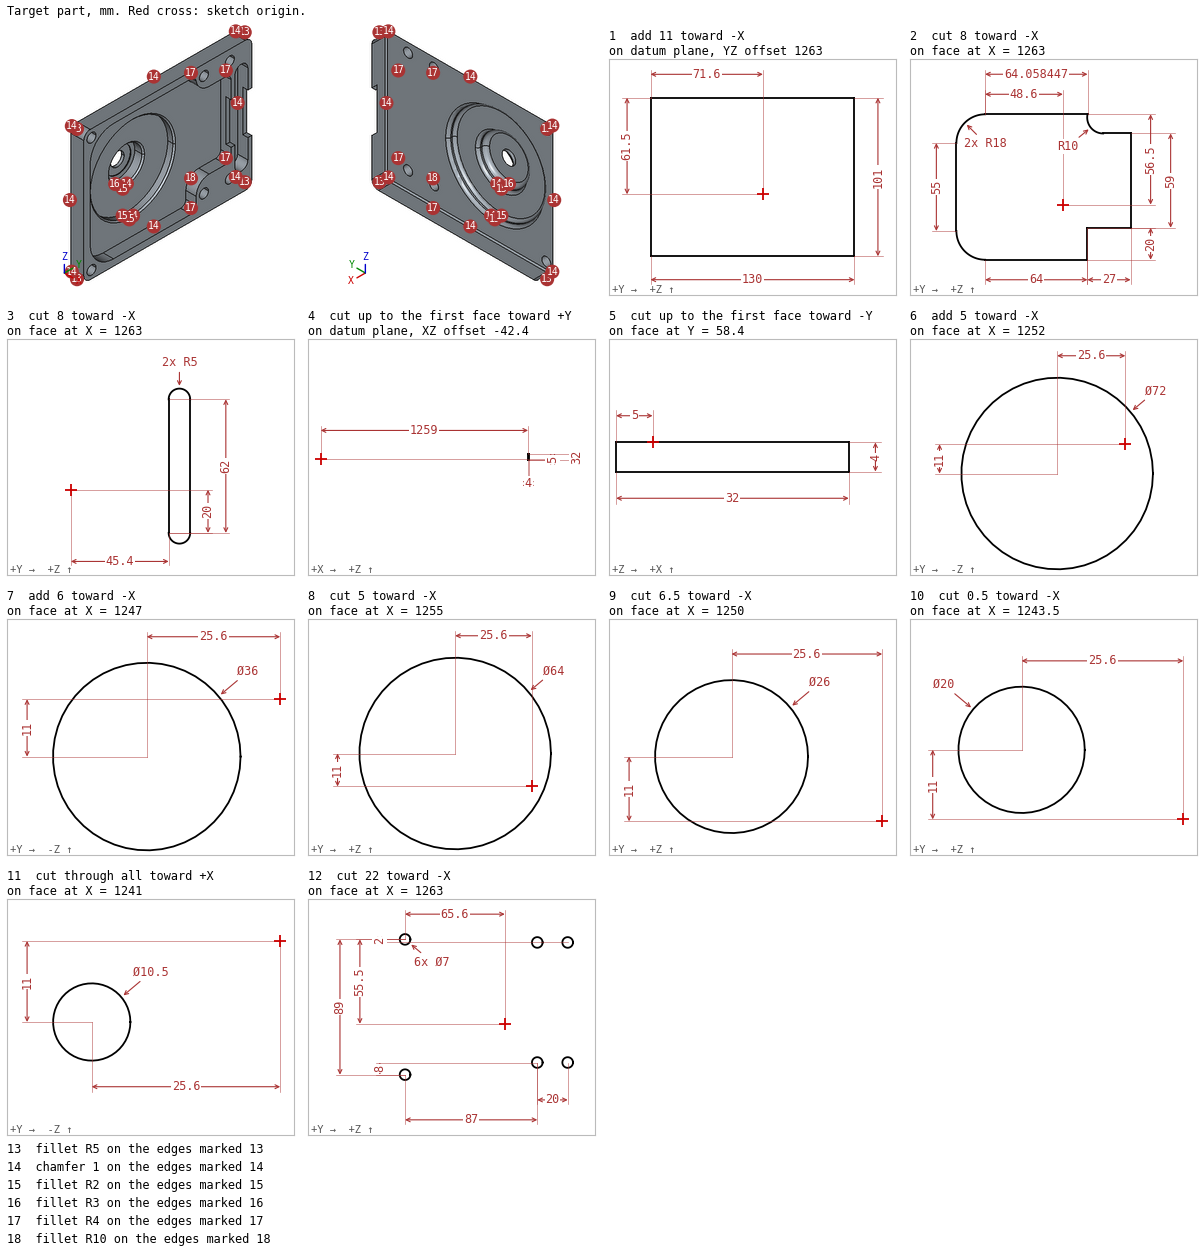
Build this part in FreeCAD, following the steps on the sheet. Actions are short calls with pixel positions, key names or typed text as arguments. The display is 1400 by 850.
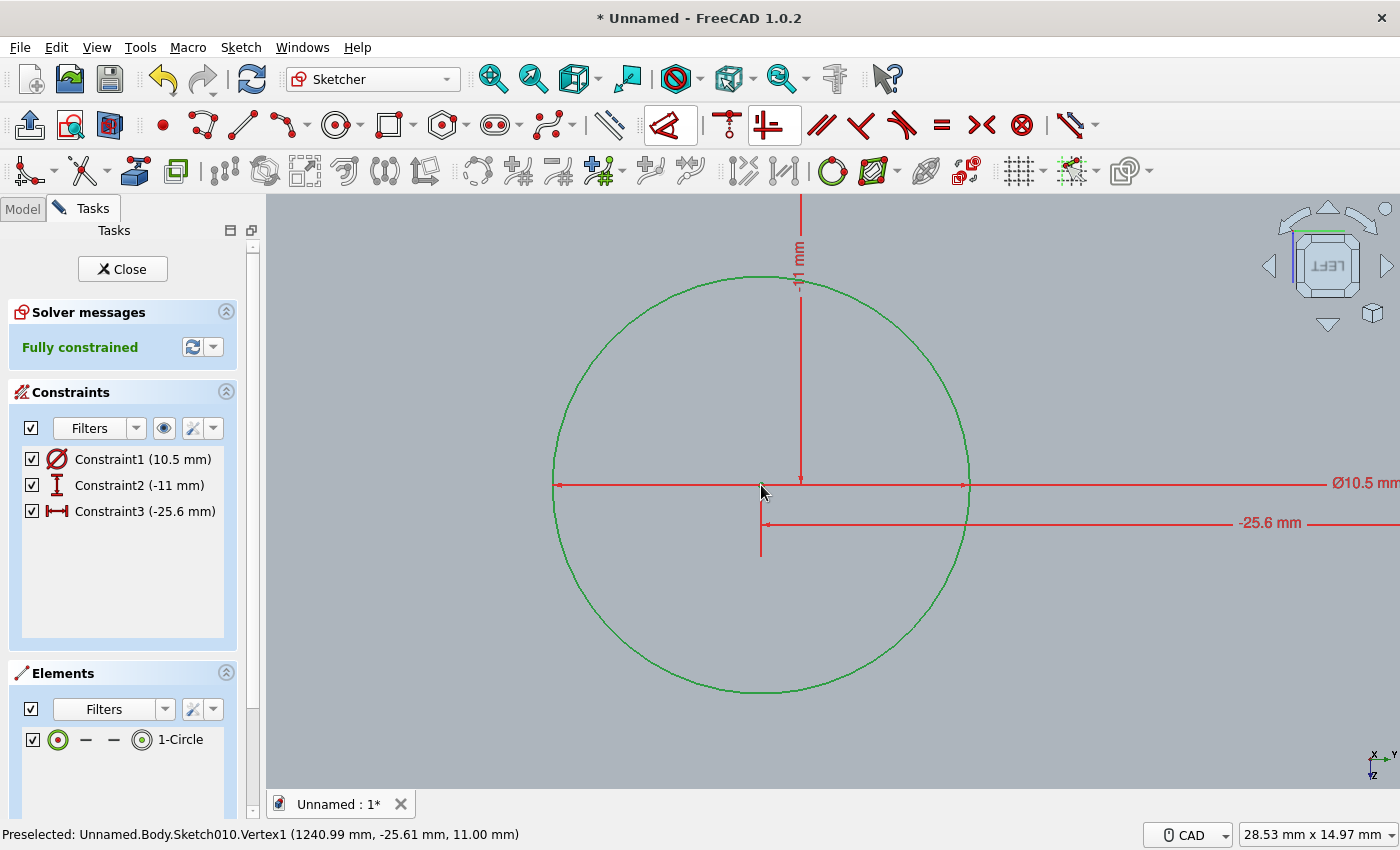
click(123, 269)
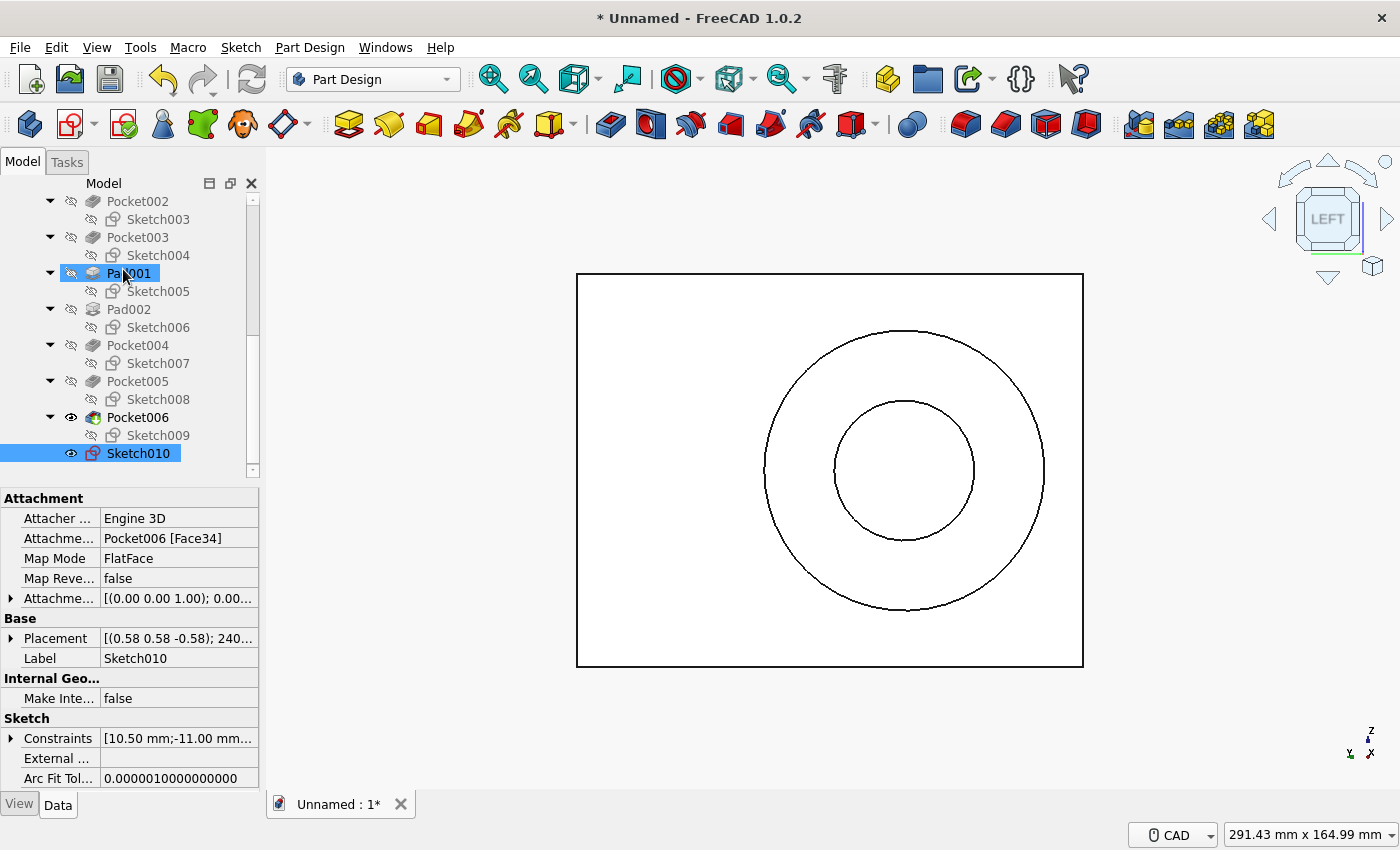
click(612, 124)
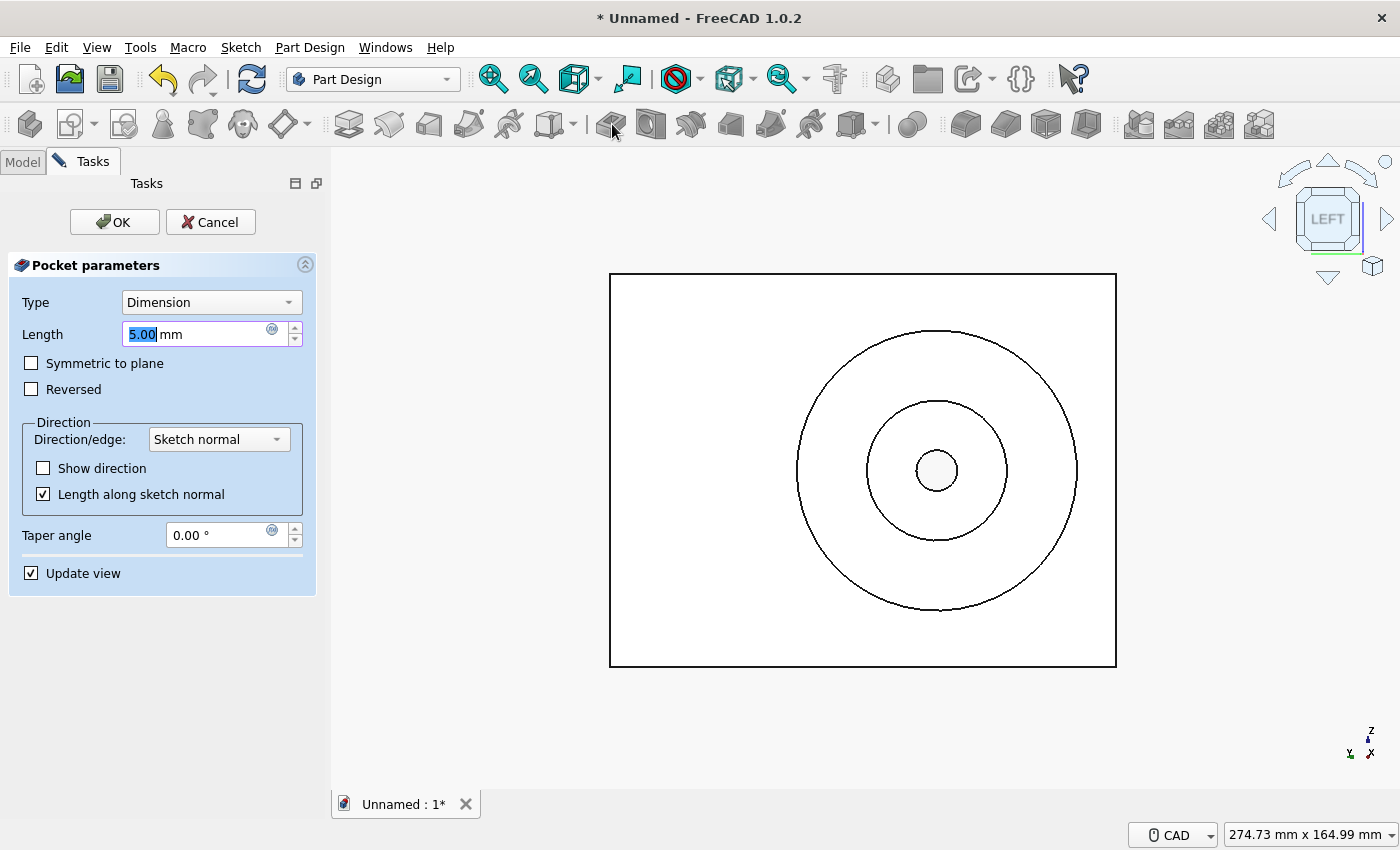
click(212, 302)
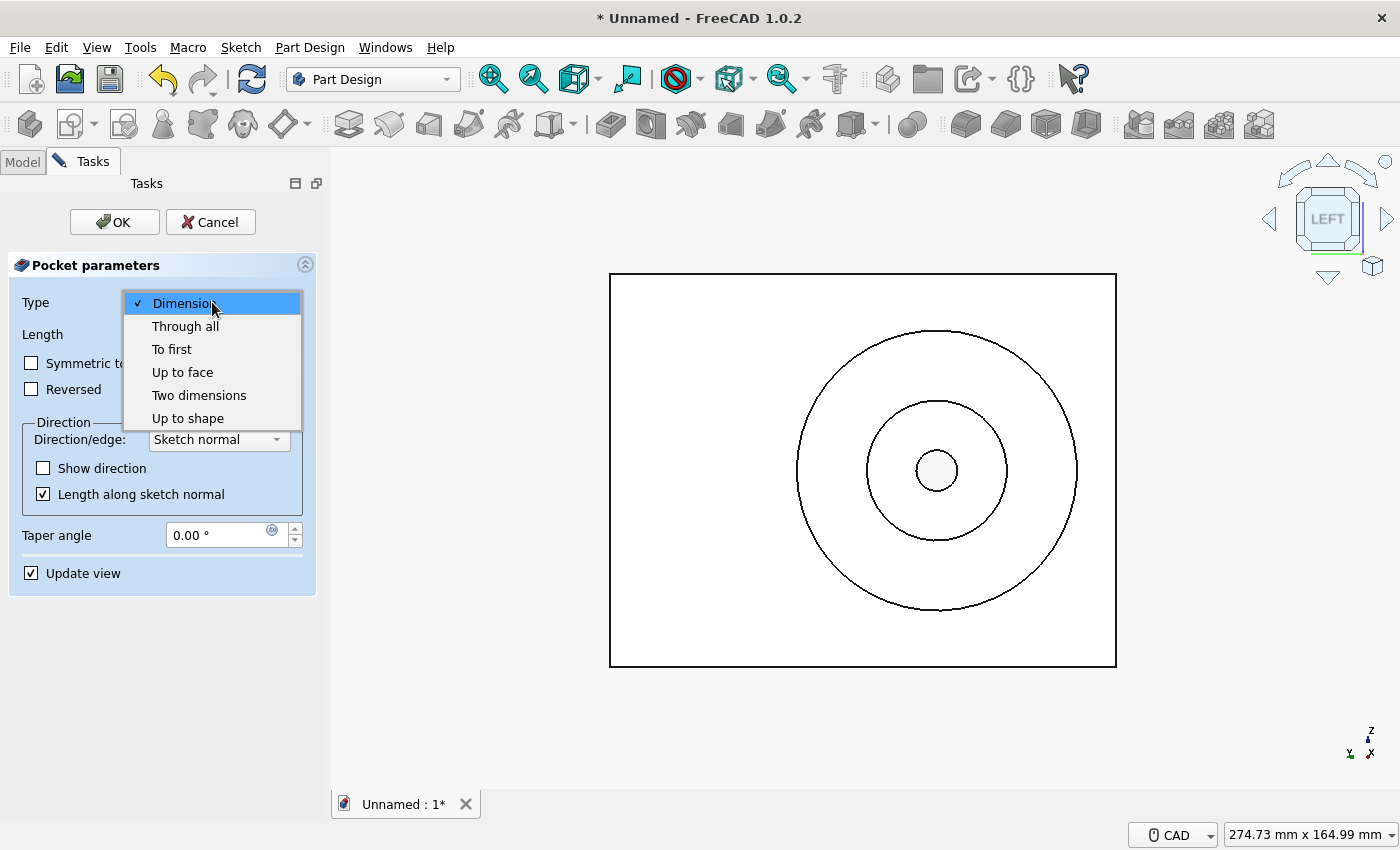
click(212, 326)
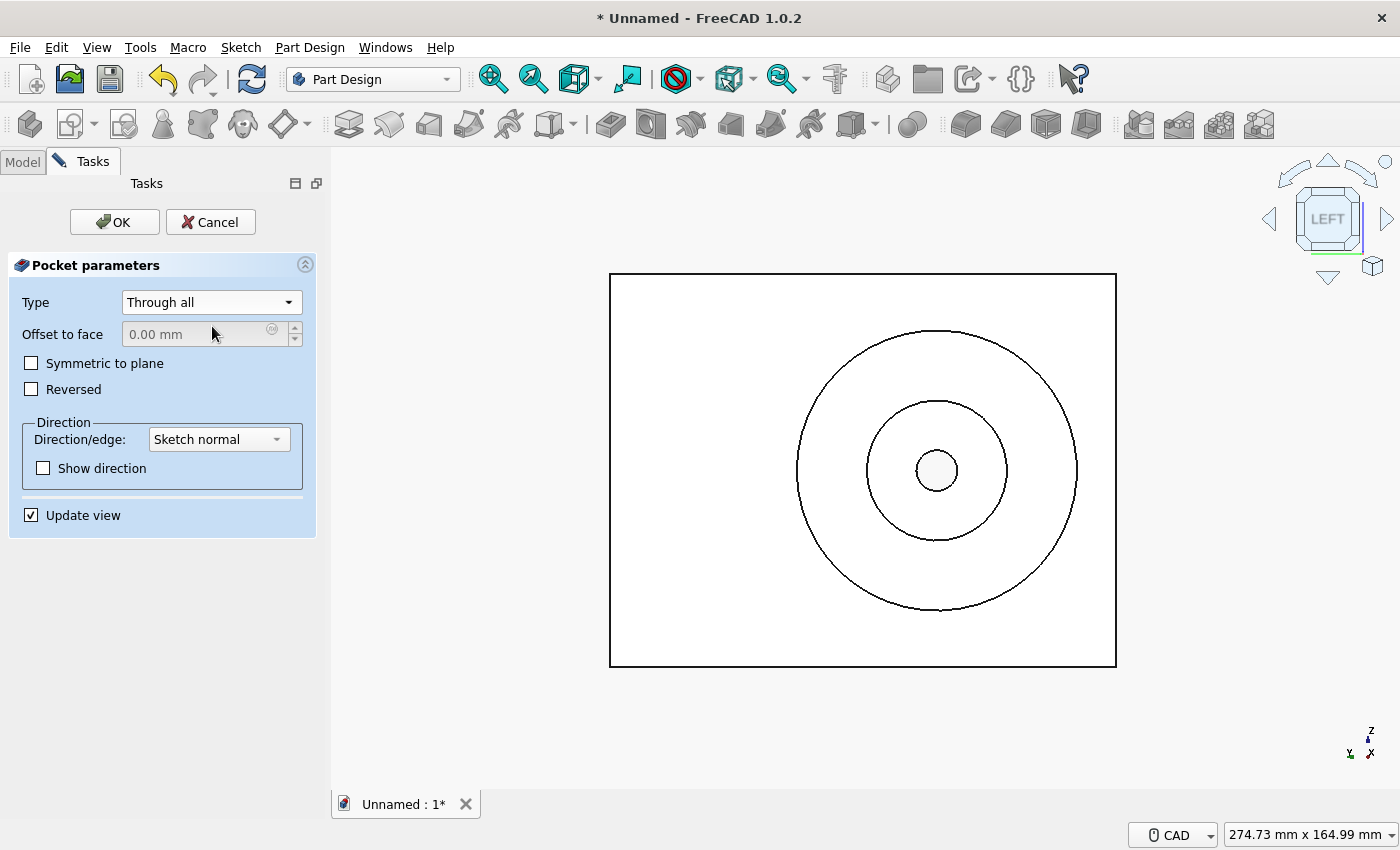
click(115, 222)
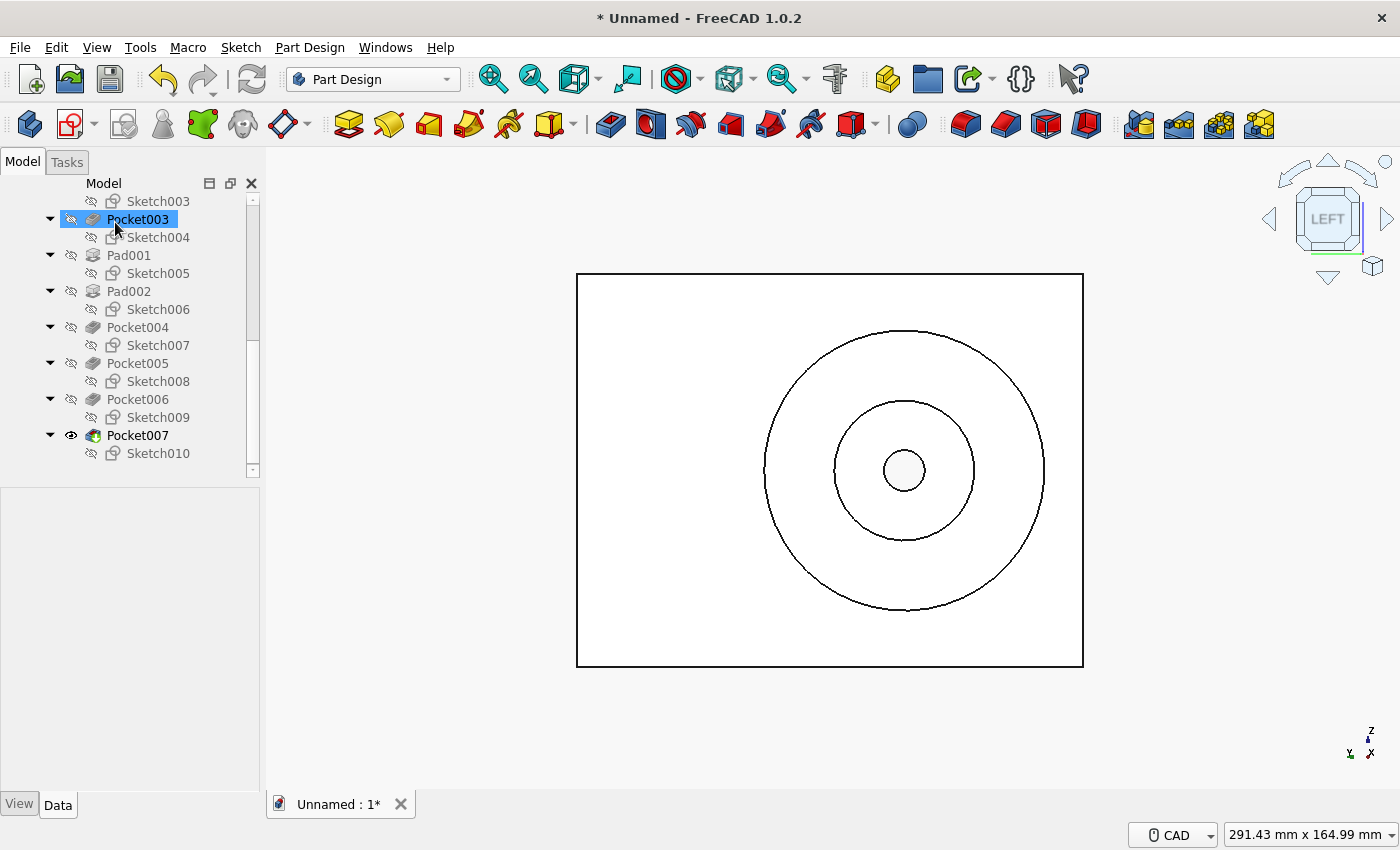
key(0)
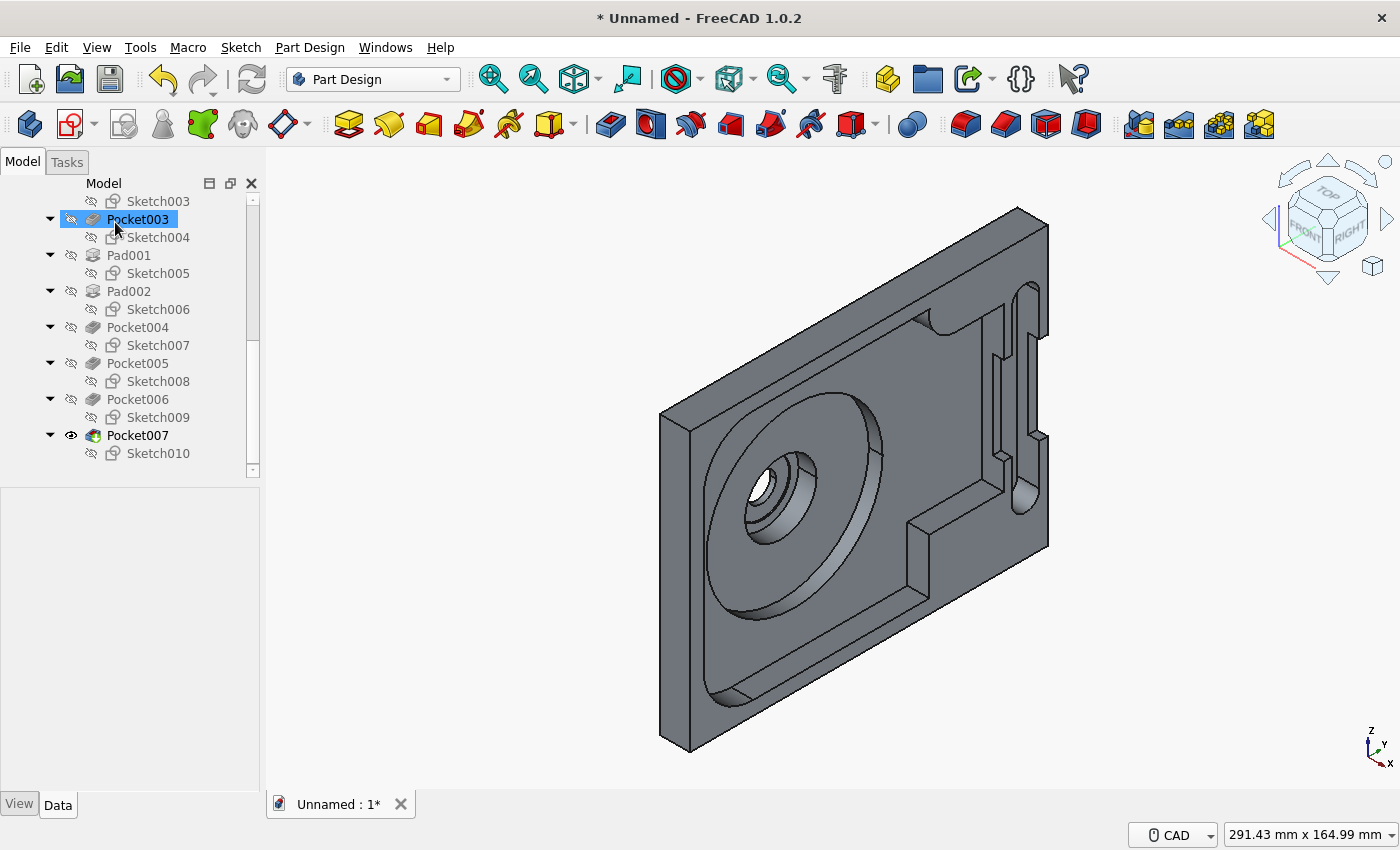
click(1022, 537)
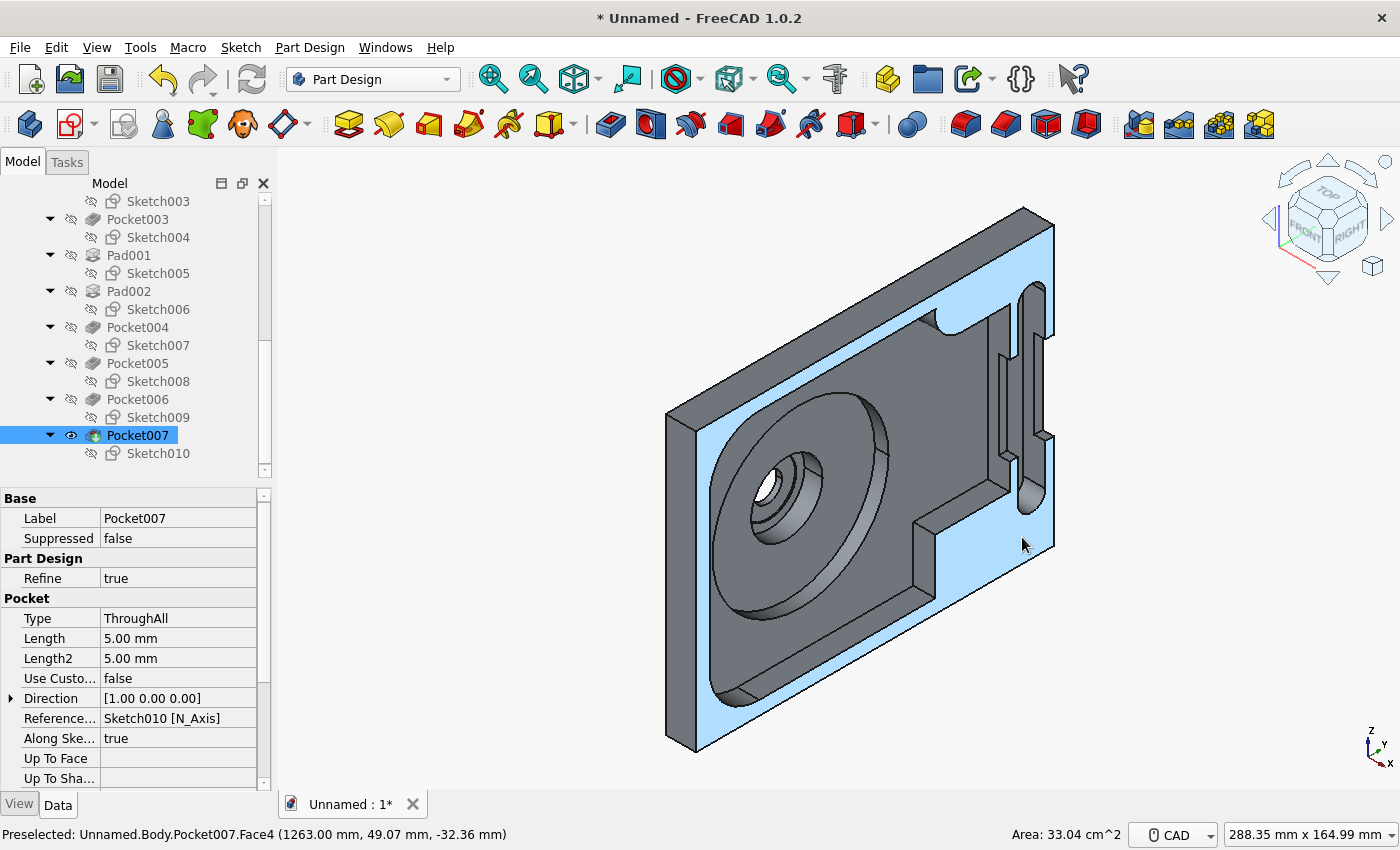
click(70, 124)